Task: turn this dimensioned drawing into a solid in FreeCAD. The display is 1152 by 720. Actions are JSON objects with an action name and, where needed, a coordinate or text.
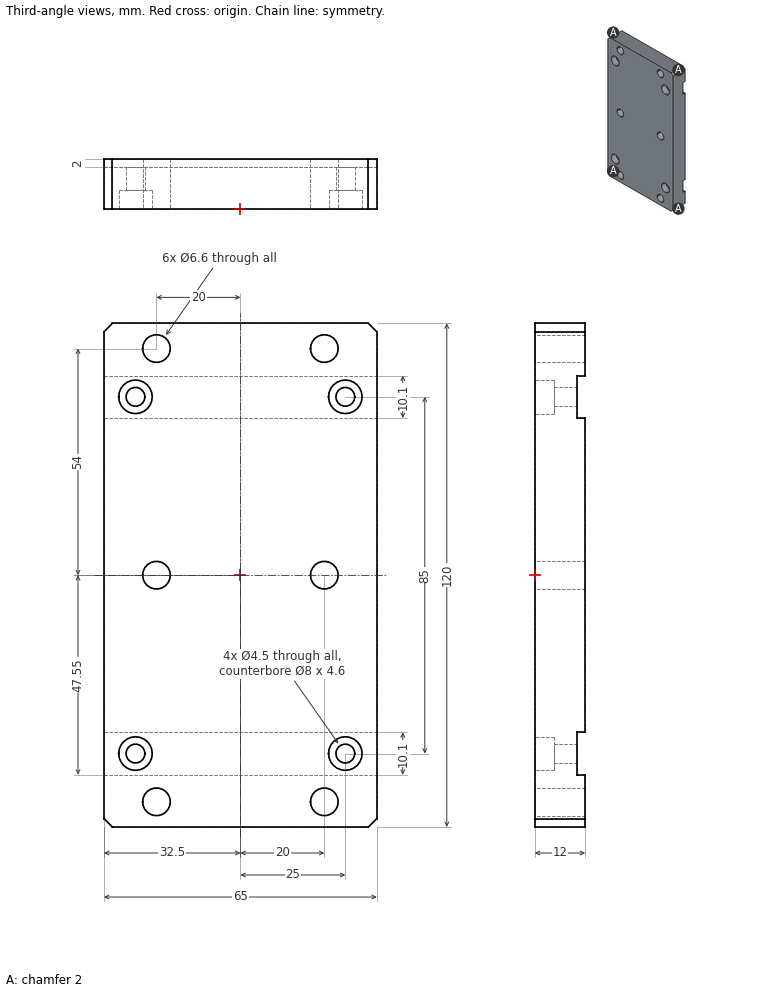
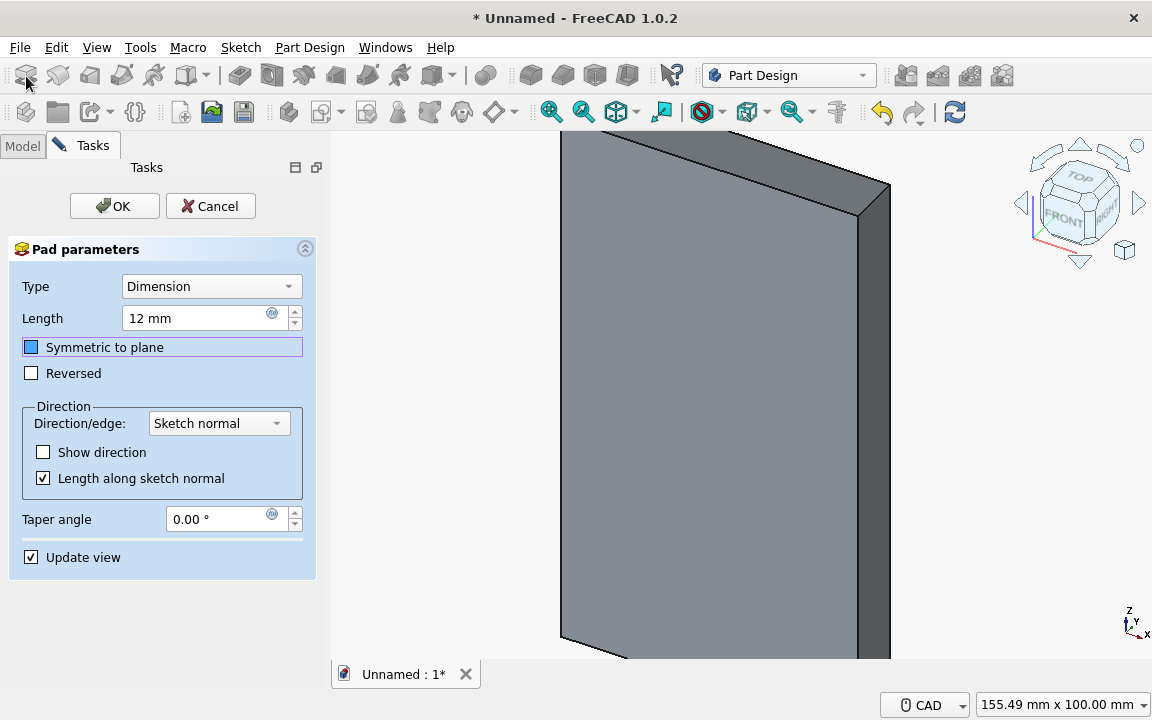
{"action": "left_click", "coordinate": [30, 373]}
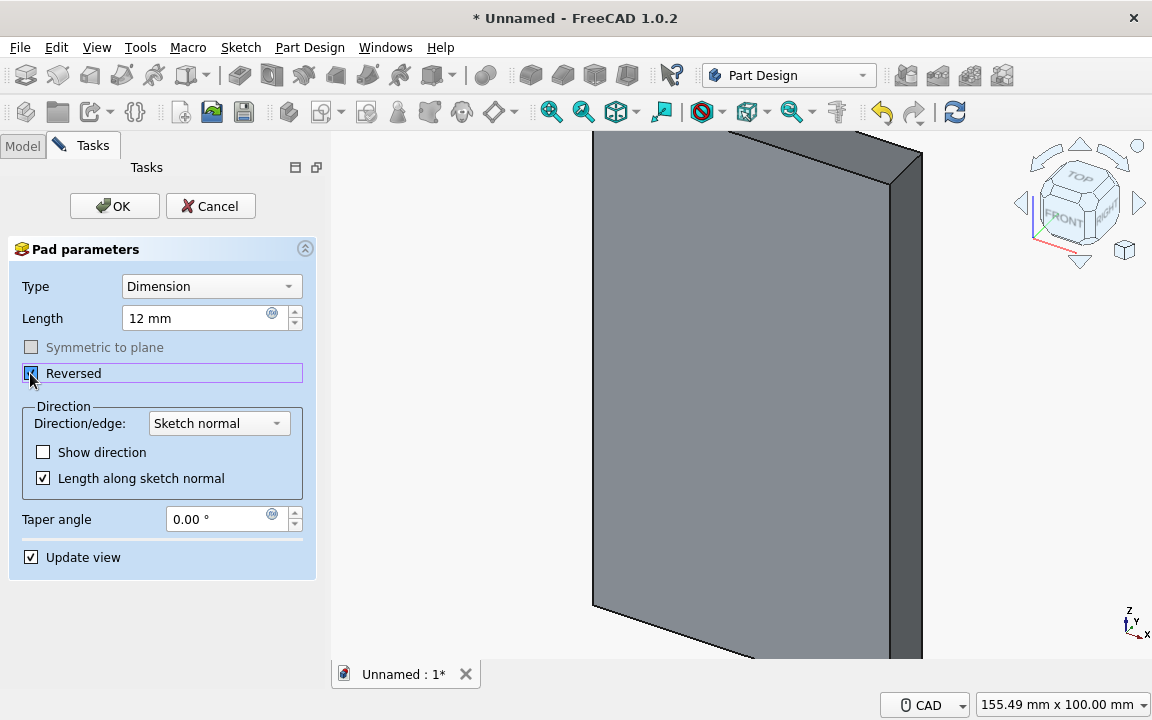
{"action": "left_click", "coordinate": [115, 206]}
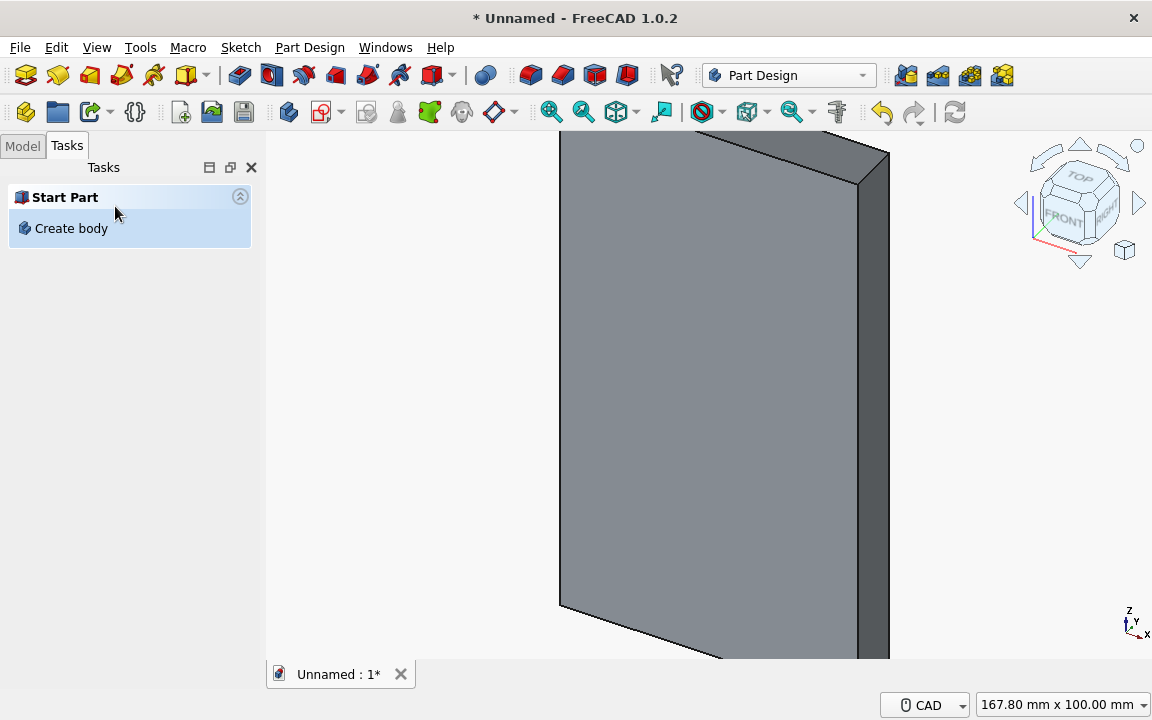
{"action": "key", "text": "v f"}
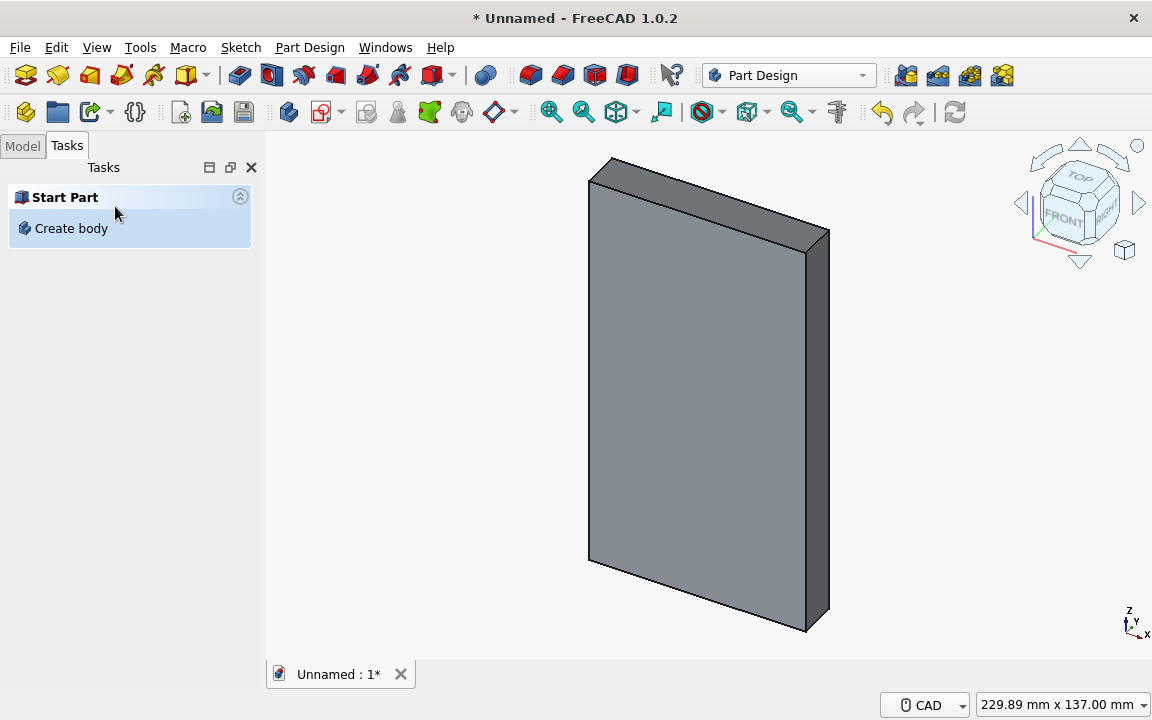
{"action": "key", "text": "4"}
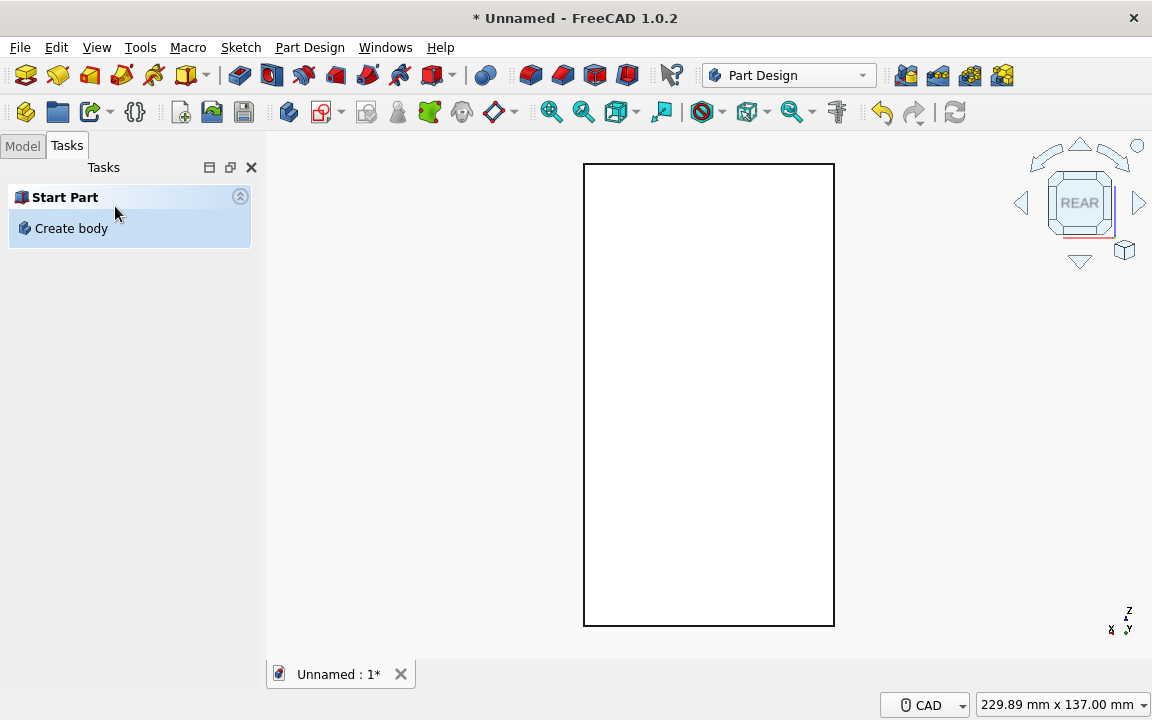
{"action": "left_click", "coordinate": [709, 328]}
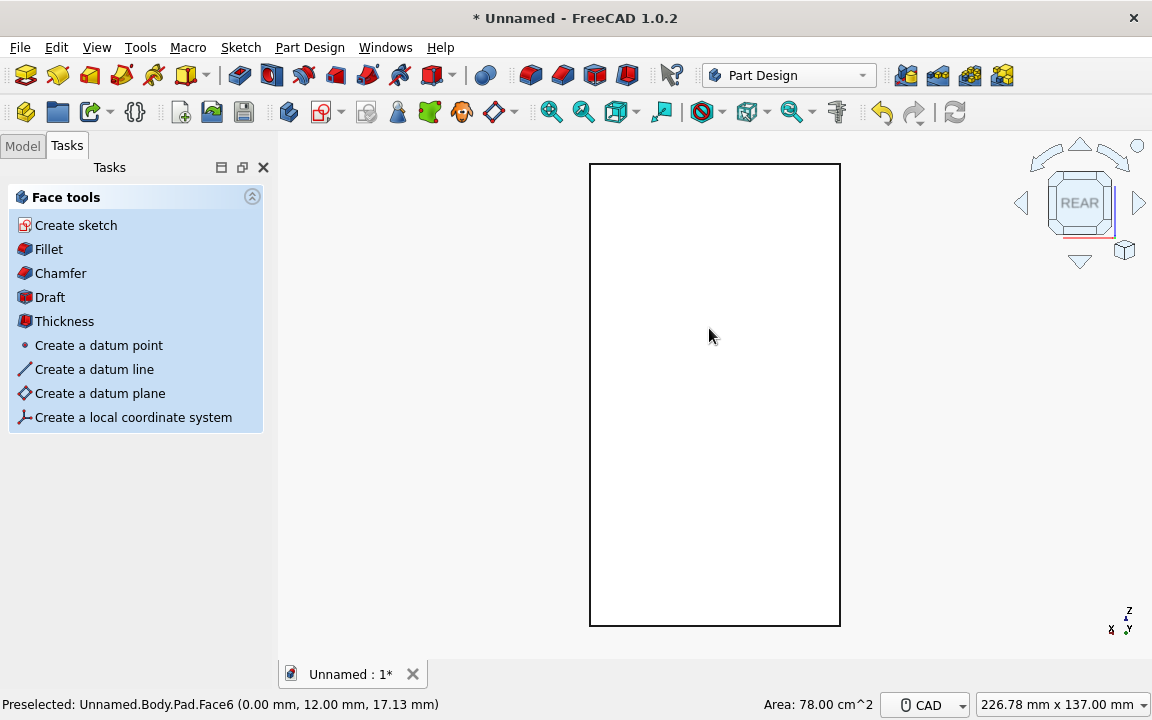
{"action": "left_click", "coordinate": [322, 112]}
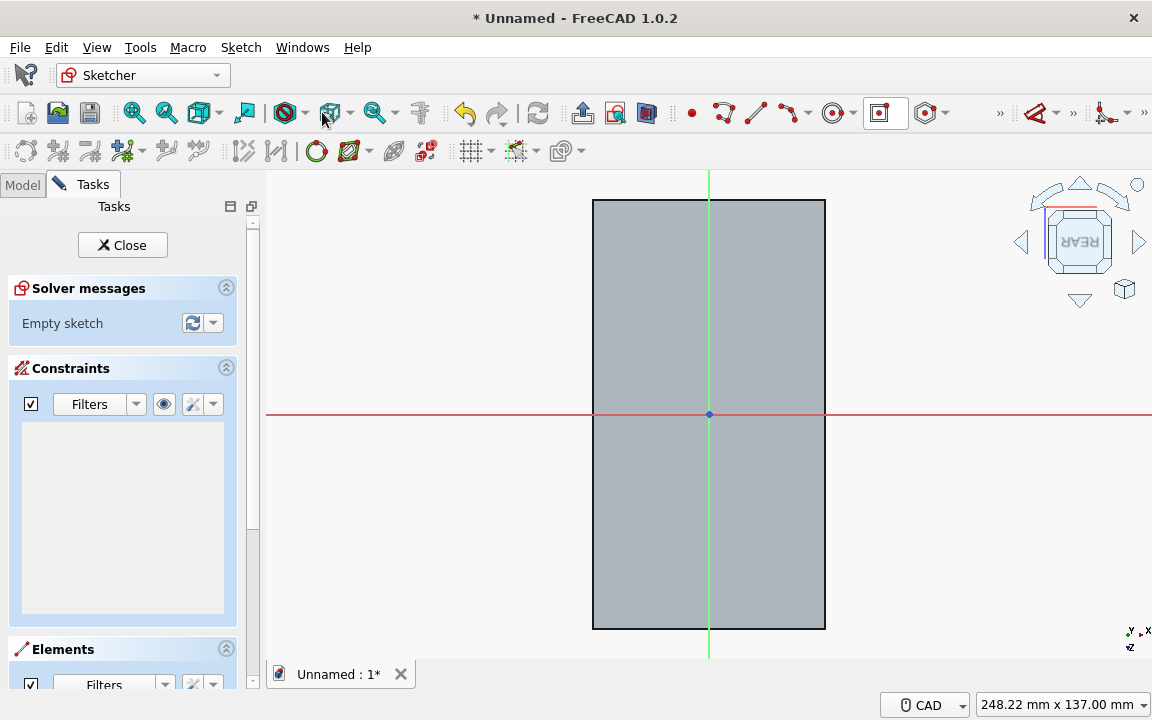
{"action": "scroll", "coordinate": [331, 414], "scroll_direction": "down", "scroll_amount": 1}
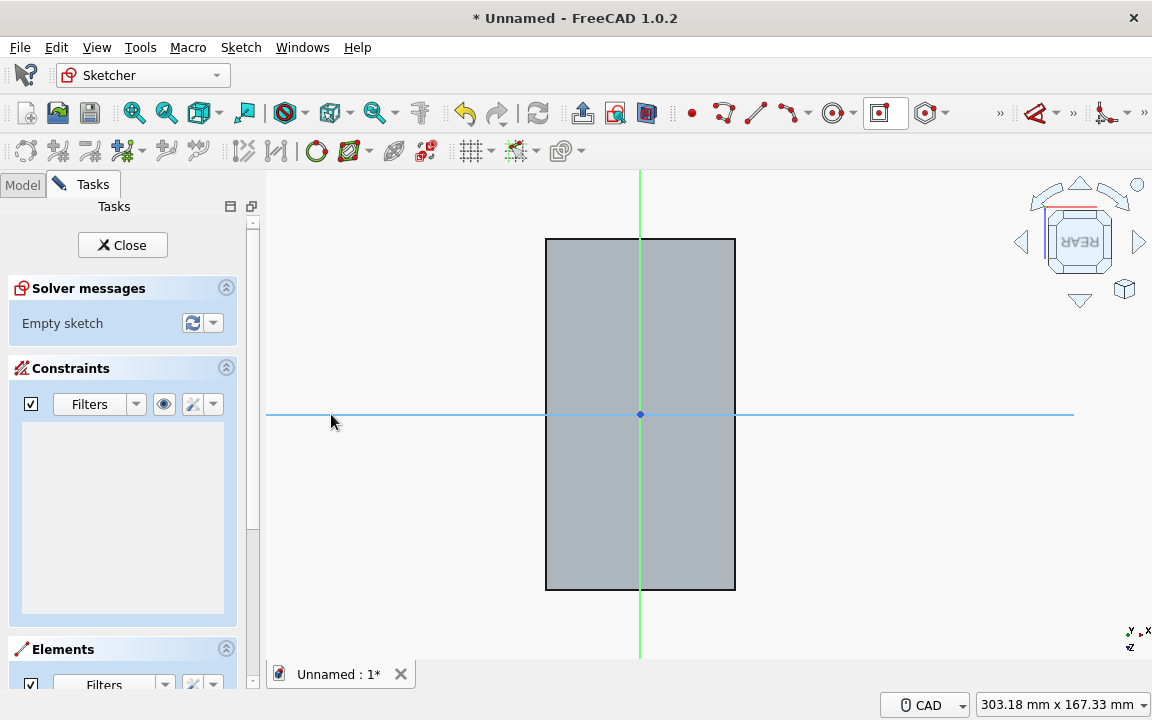
{"action": "left_click", "coordinate": [834, 114]}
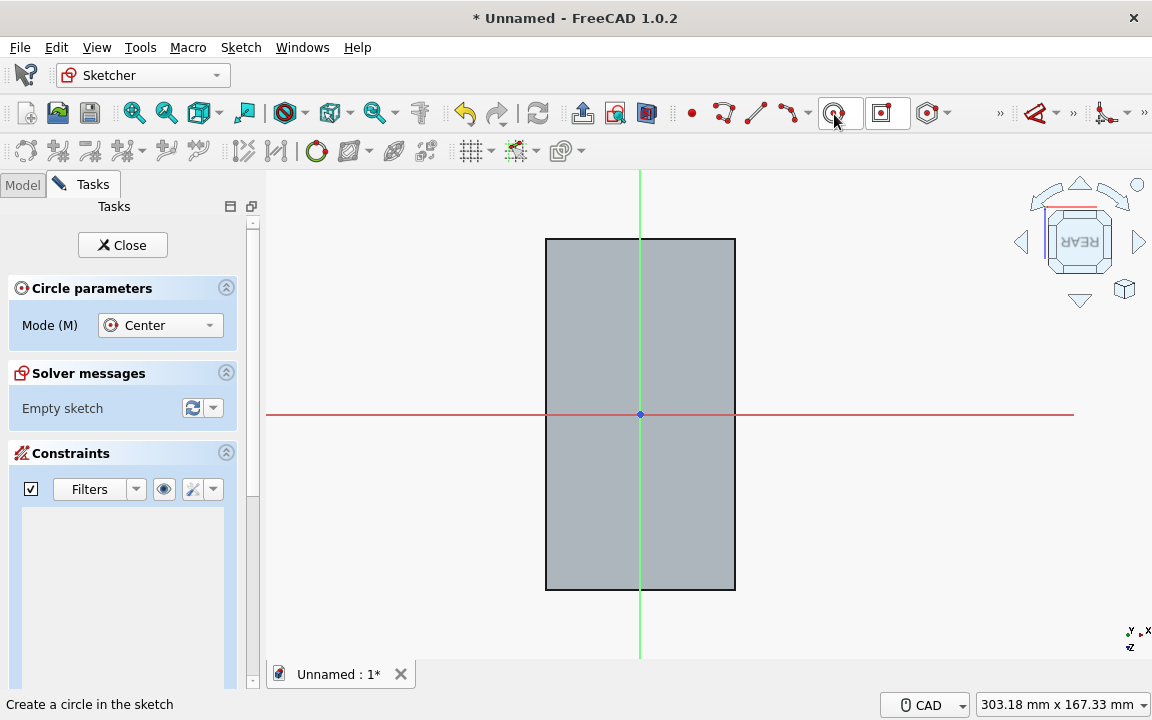
{"action": "scroll", "coordinate": [582, 572], "scroll_direction": "up", "scroll_amount": 5}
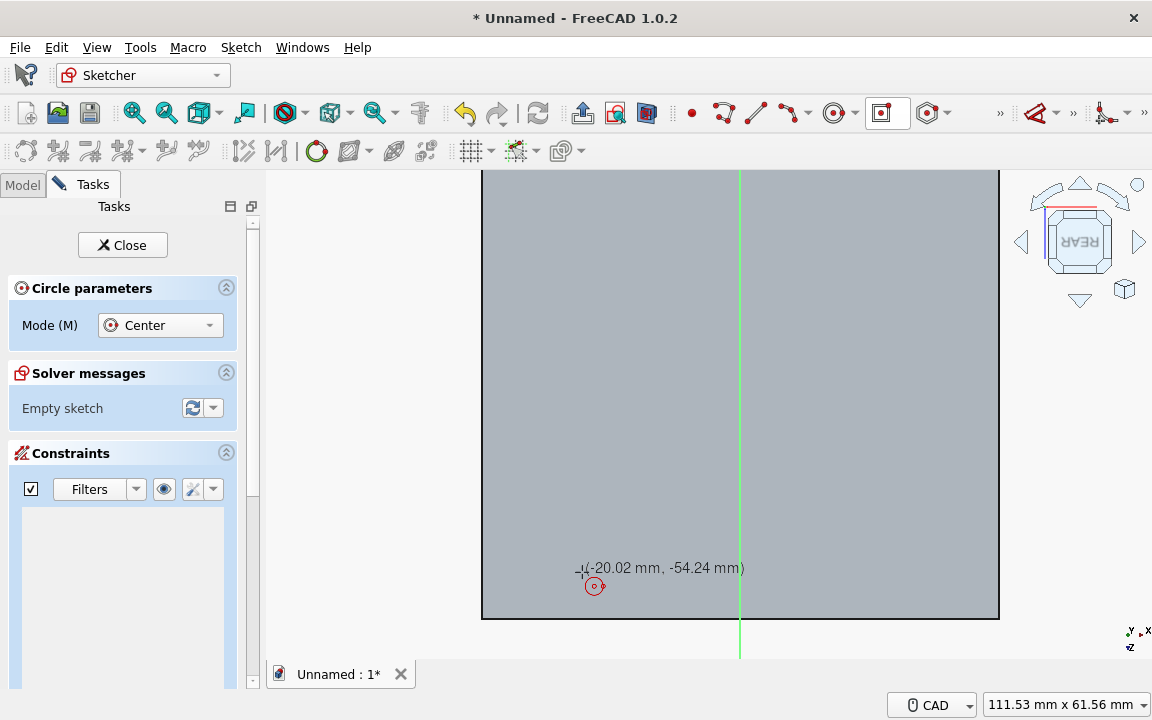
{"action": "left_click", "coordinate": [582, 571]}
{"action": "mouse_move", "coordinate": [600, 553]}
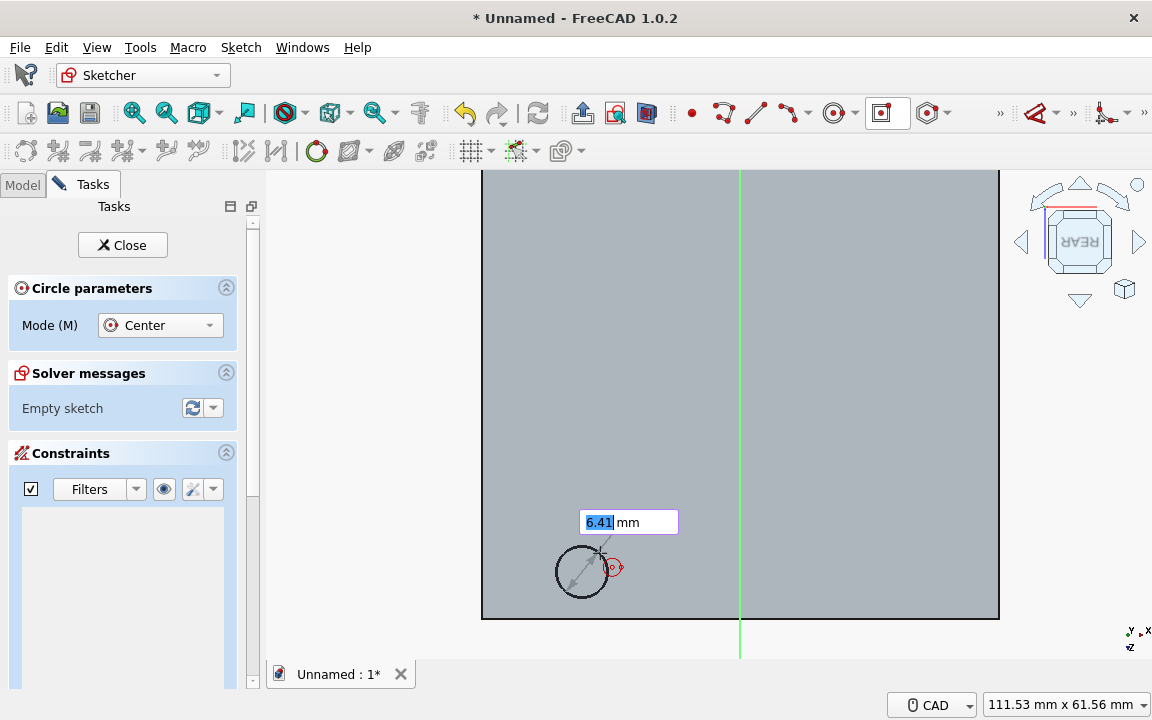
{"action": "type", "text": "6.6"}
{"action": "key", "text": "Return"}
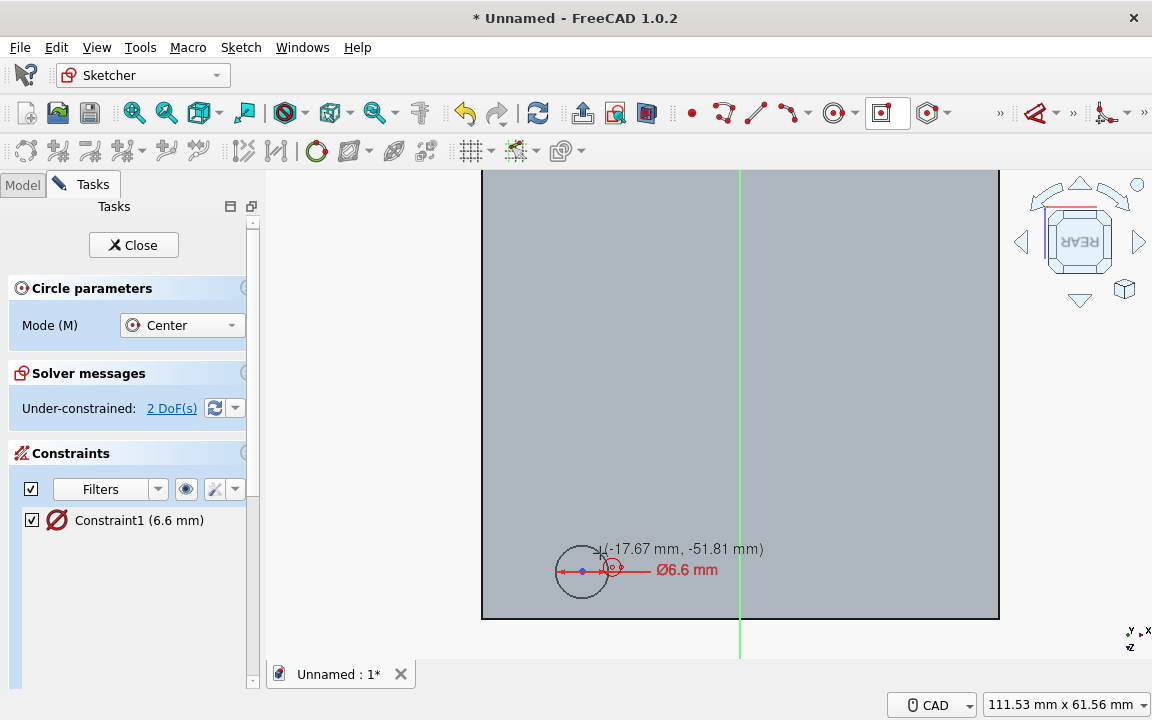
{"action": "left_click", "coordinate": [899, 571]}
{"action": "mouse_move", "coordinate": [918, 553]}